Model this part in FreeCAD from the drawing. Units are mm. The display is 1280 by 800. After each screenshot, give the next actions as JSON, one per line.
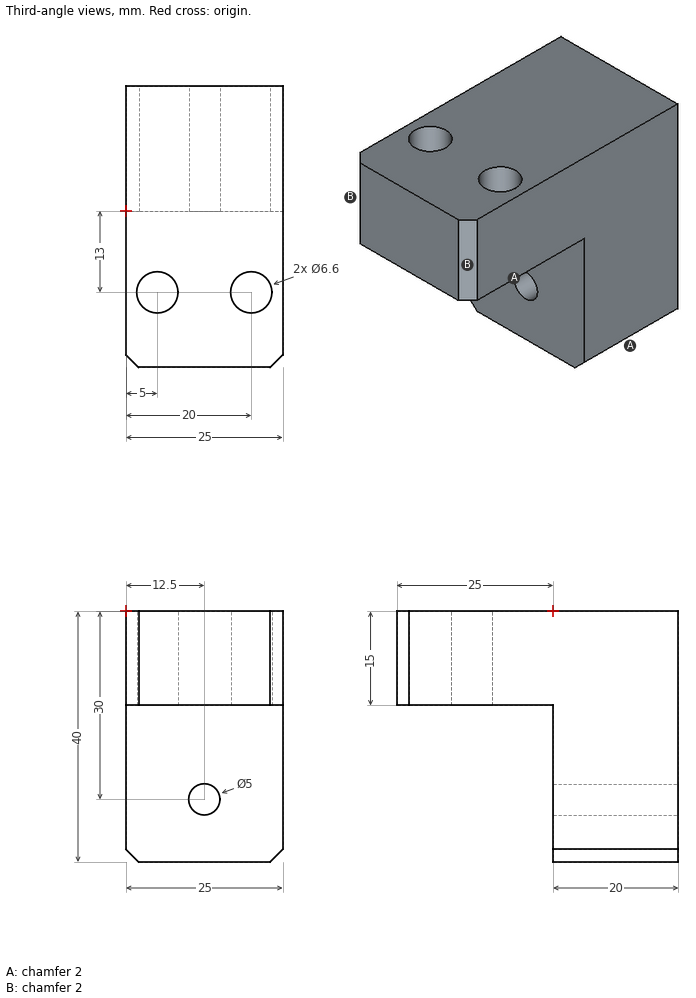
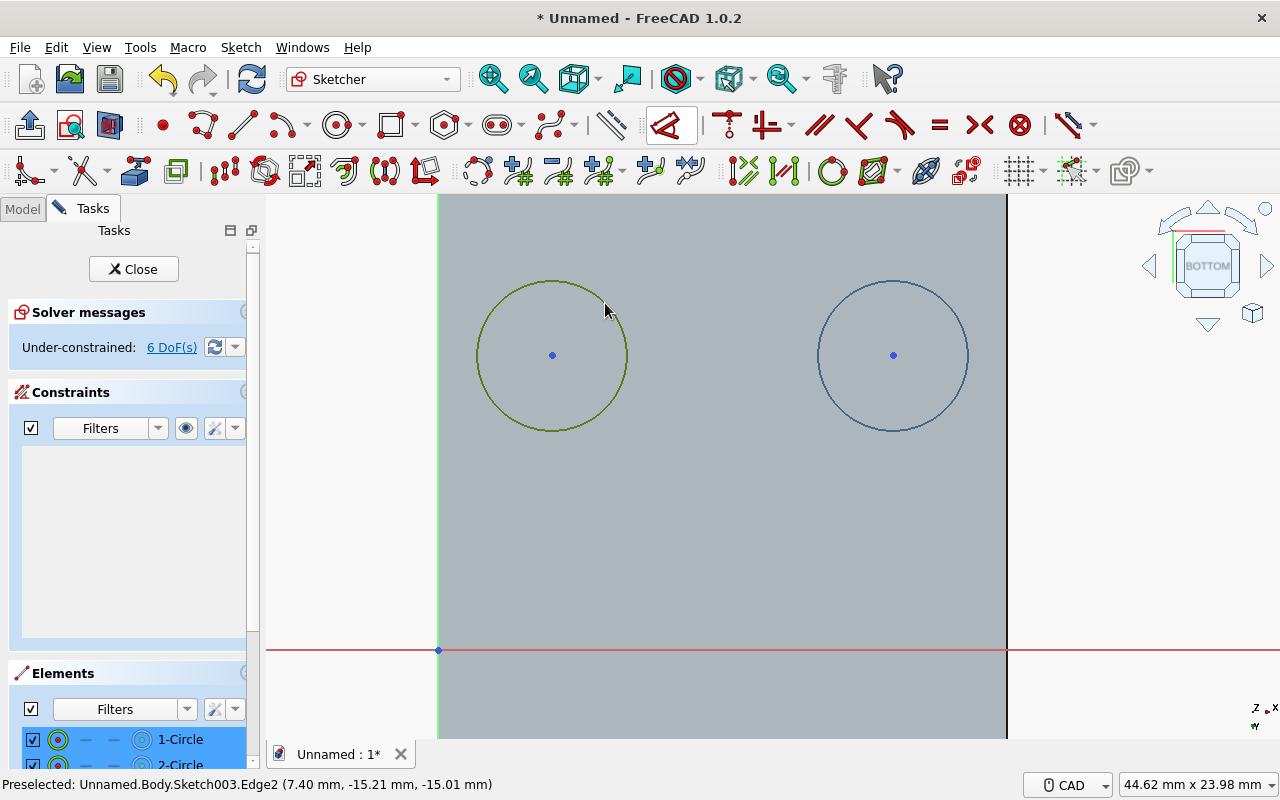
{"action": "key", "text": "e"}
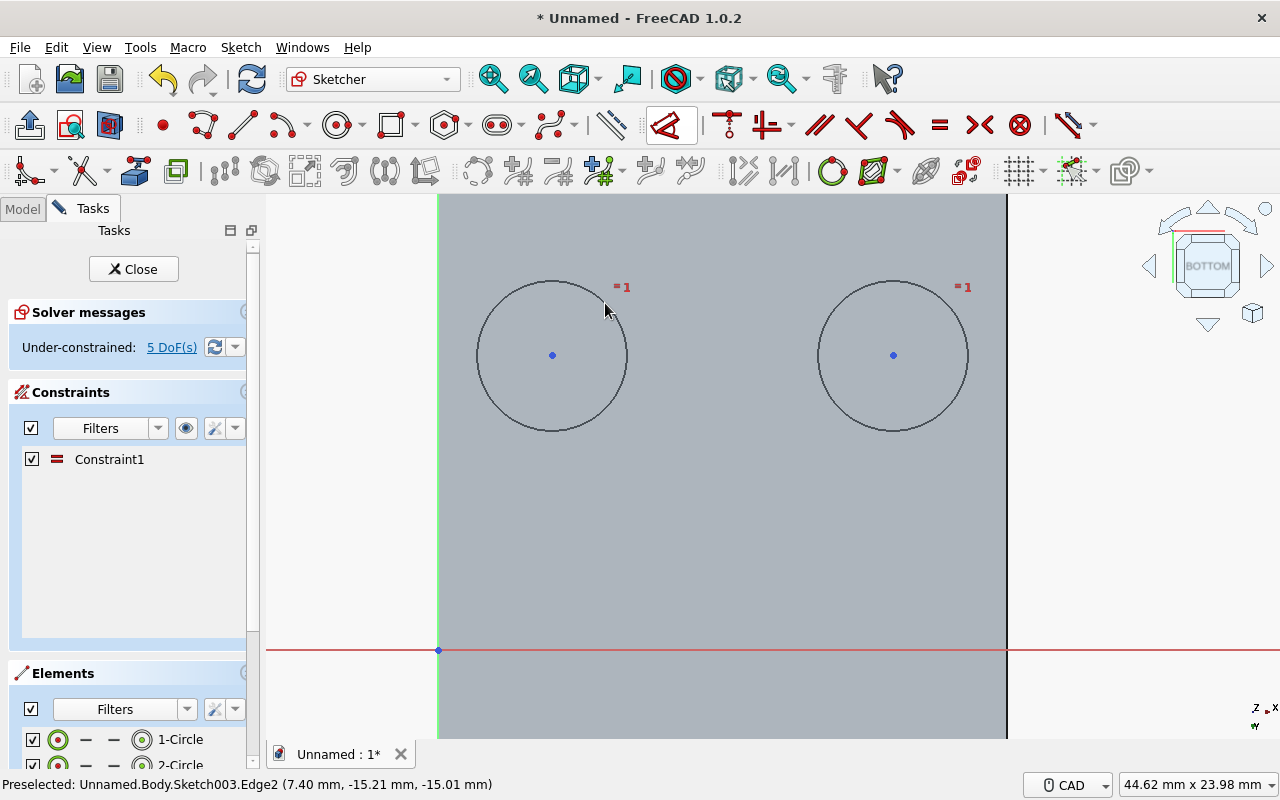
{"action": "left_click", "coordinate": [893, 356]}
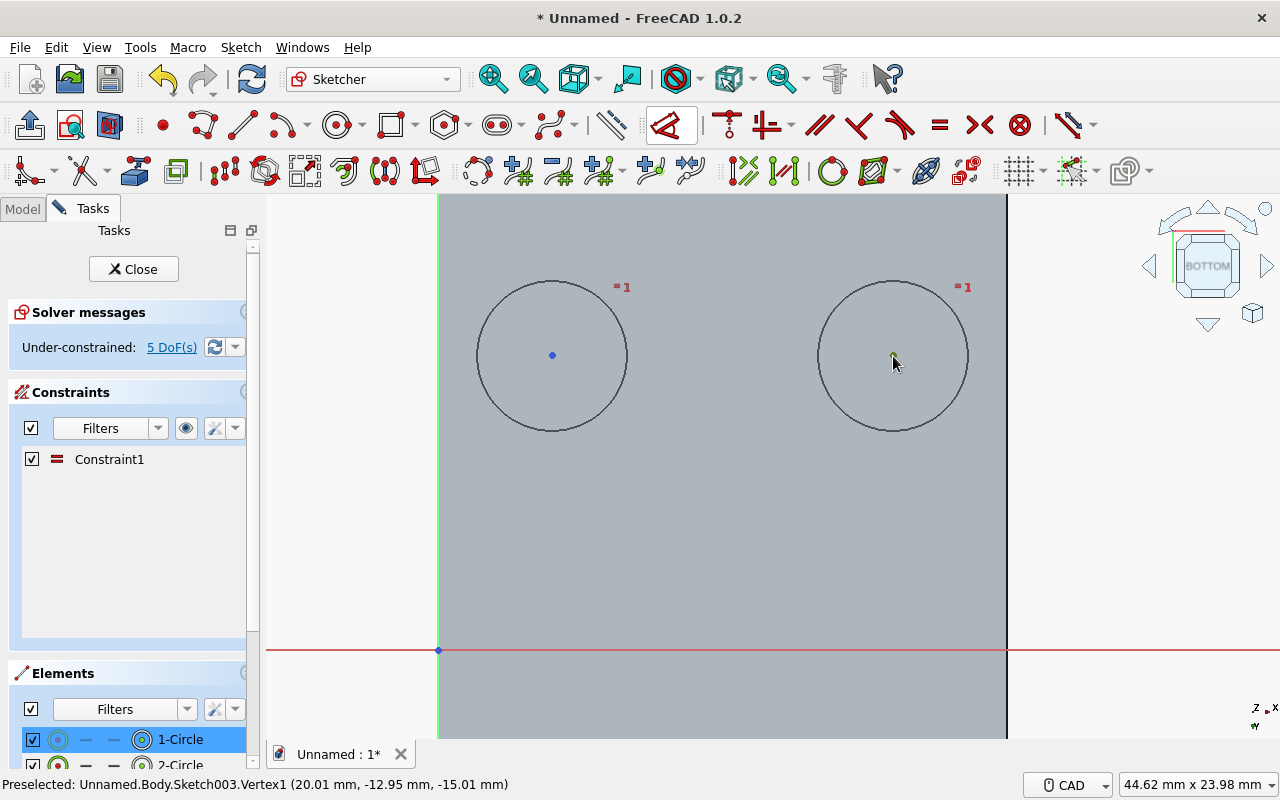
{"action": "left_click", "coordinate": [552, 356]}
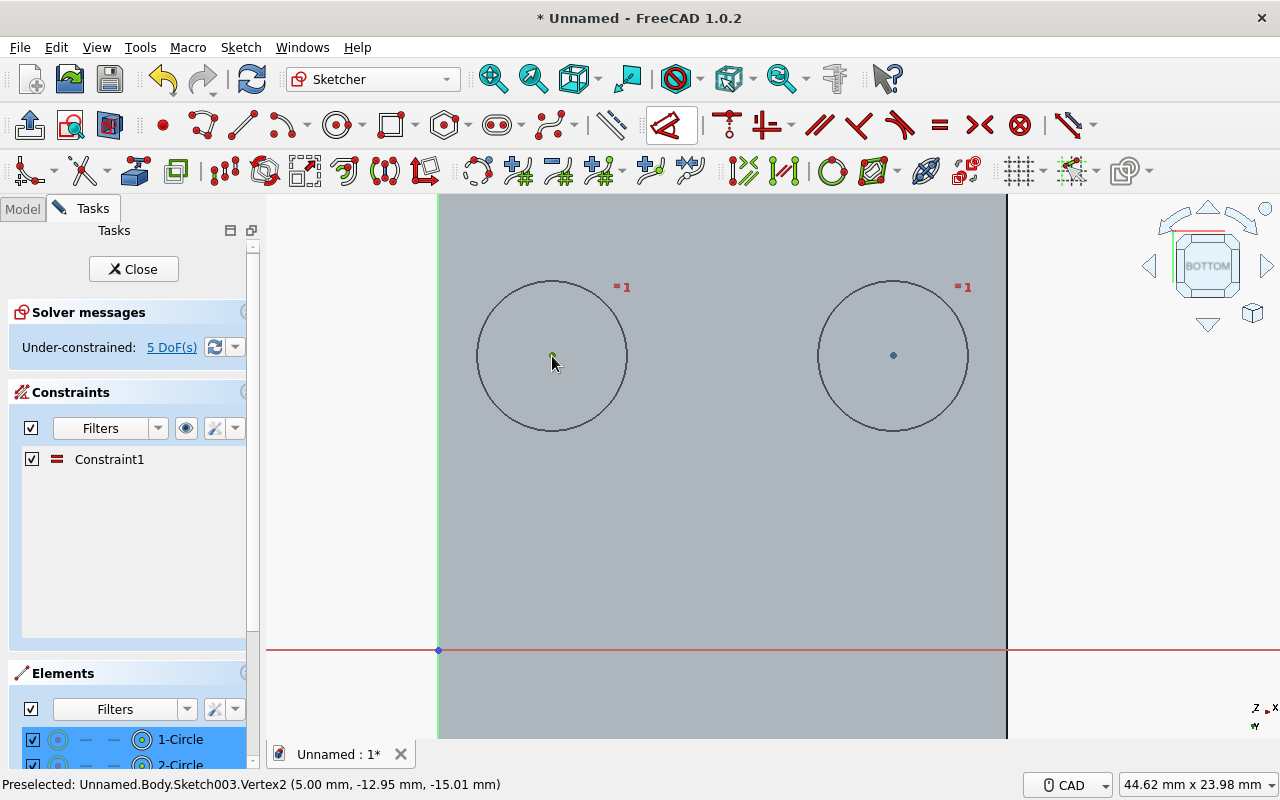
{"action": "key", "text": "h"}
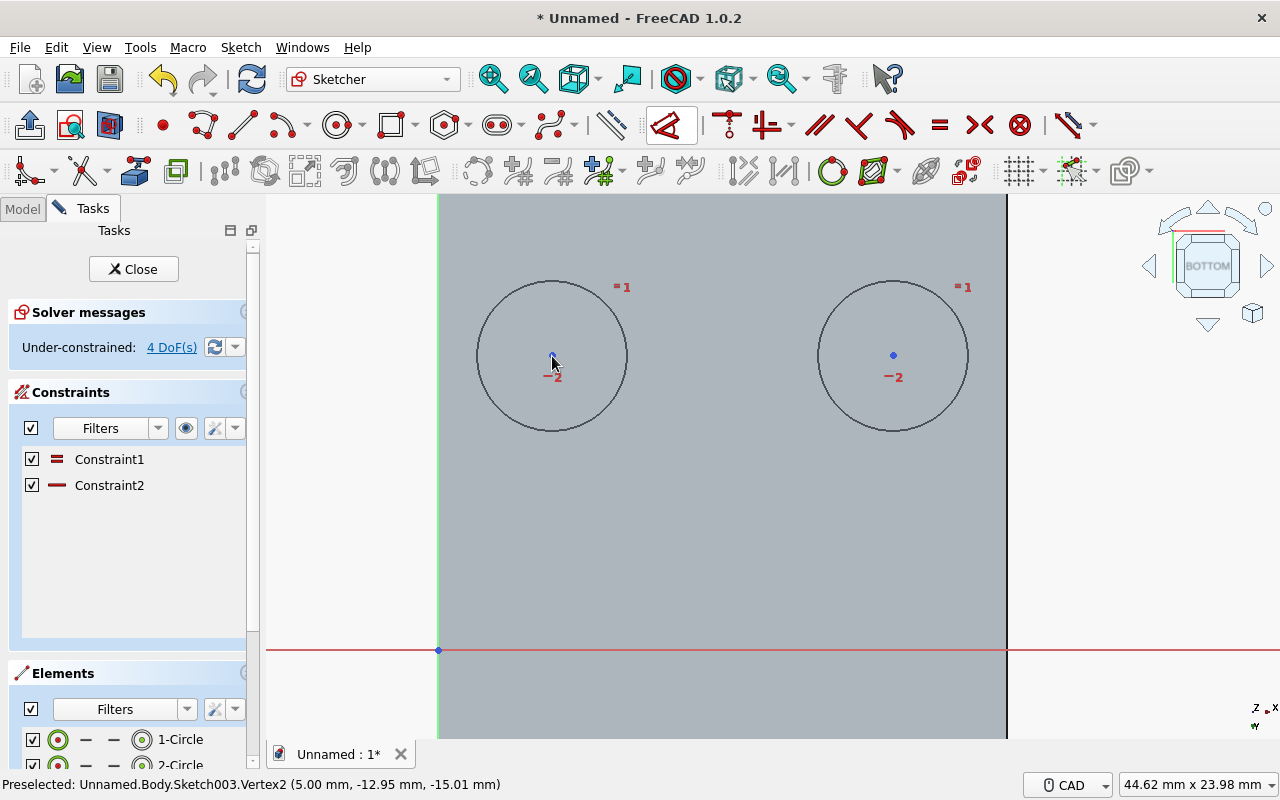
{"action": "left_click", "coordinate": [946, 303]}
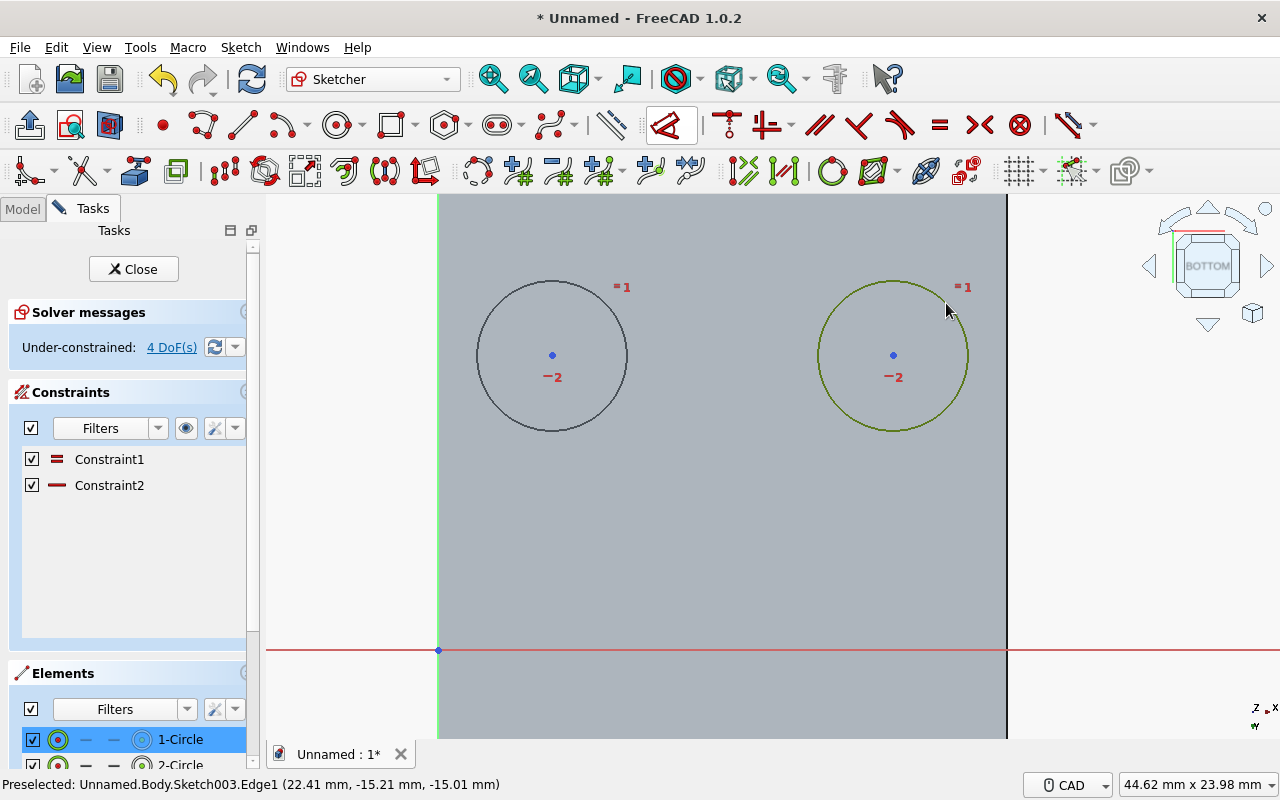
{"action": "key", "text": "k o"}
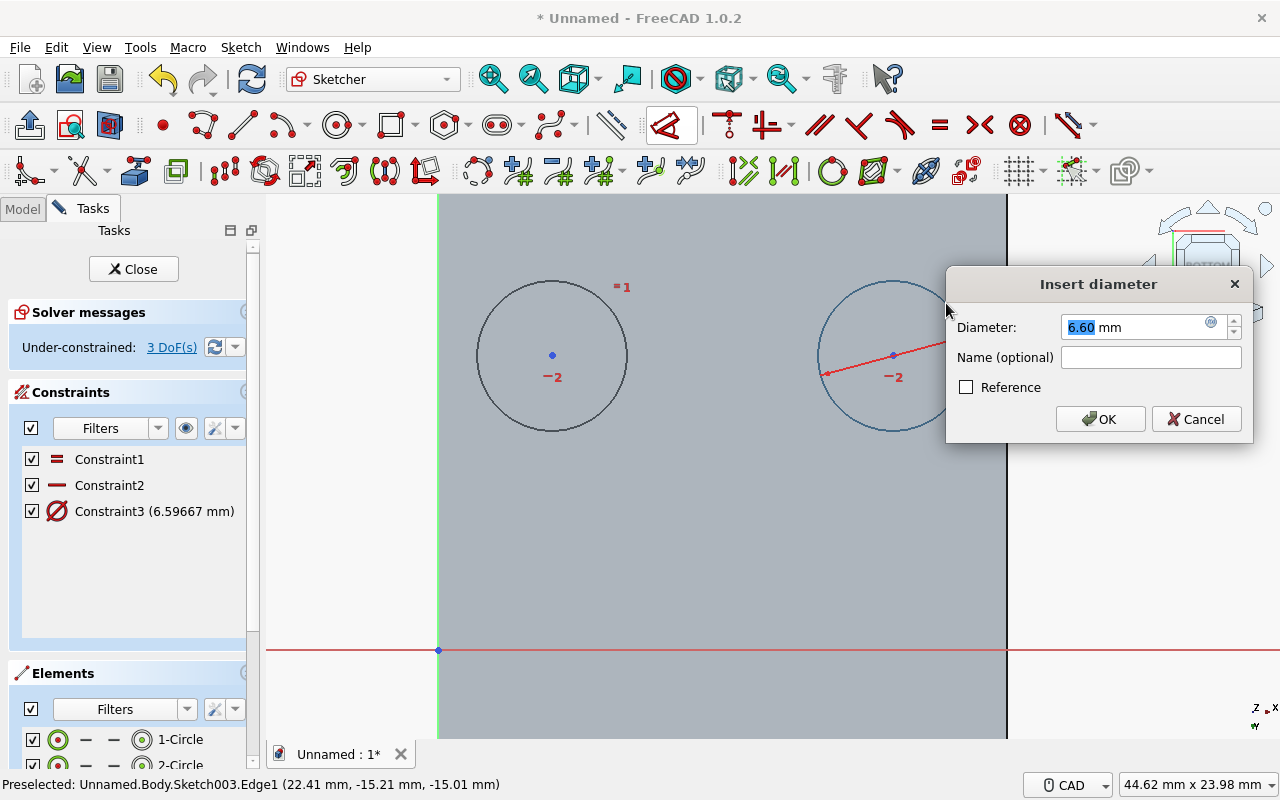
{"action": "type", "text": "6.6"}
{"action": "key", "text": "Return"}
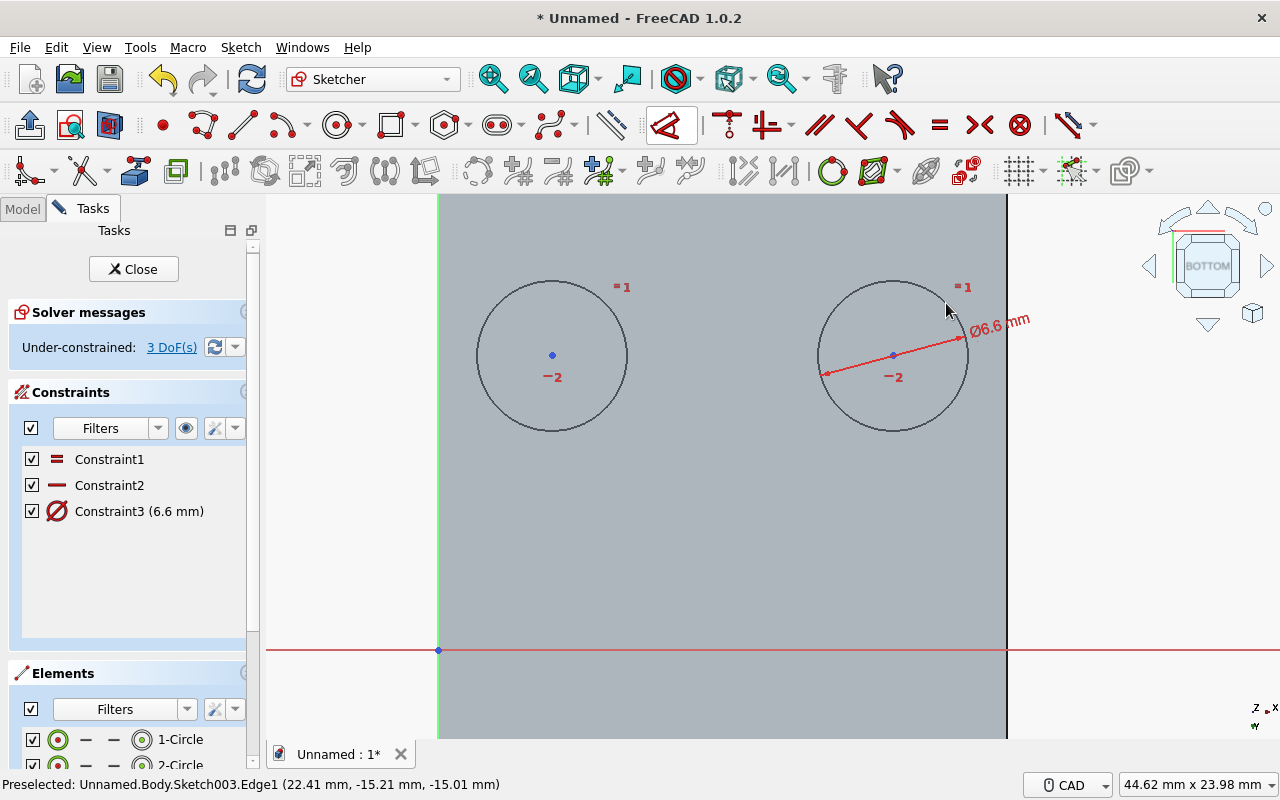
{"action": "left_click", "coordinate": [552, 356]}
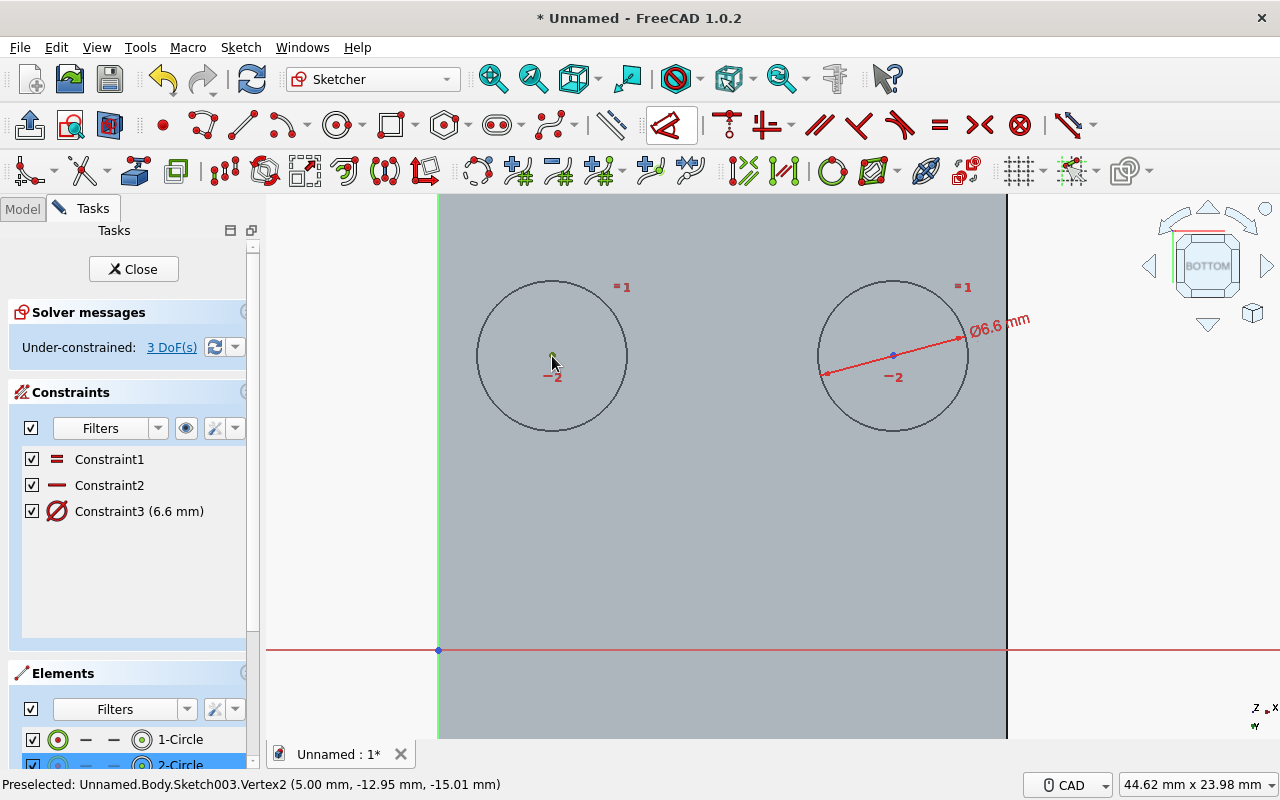
{"action": "key", "text": "l"}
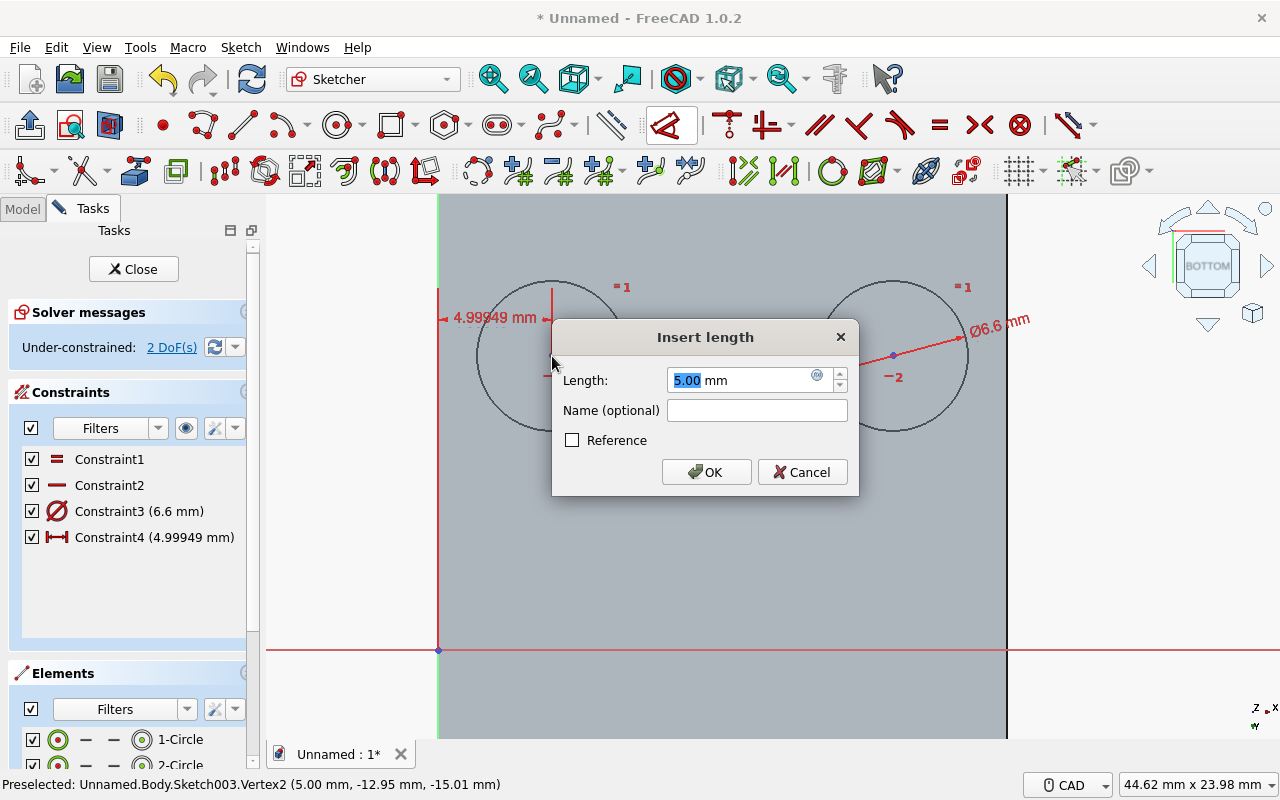
{"action": "type", "text": "5"}
{"action": "key", "text": "Return"}